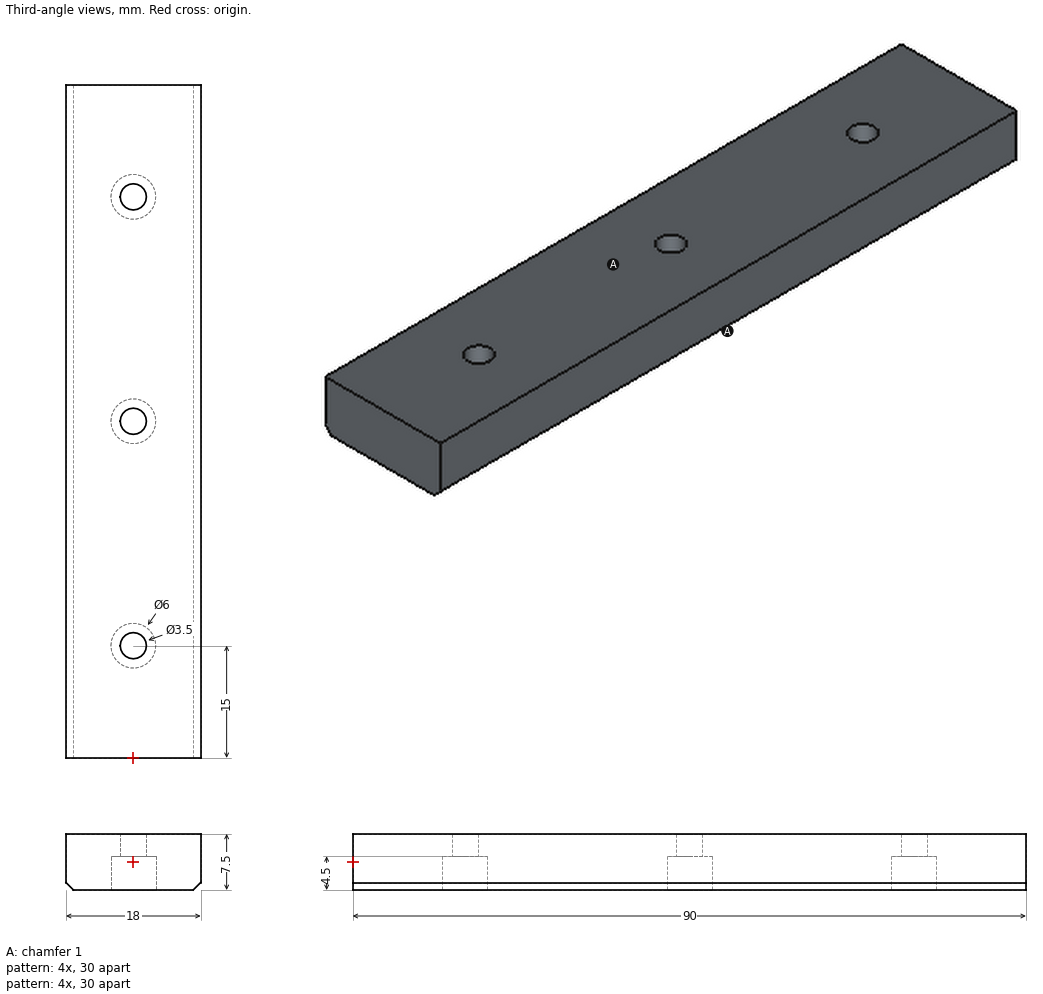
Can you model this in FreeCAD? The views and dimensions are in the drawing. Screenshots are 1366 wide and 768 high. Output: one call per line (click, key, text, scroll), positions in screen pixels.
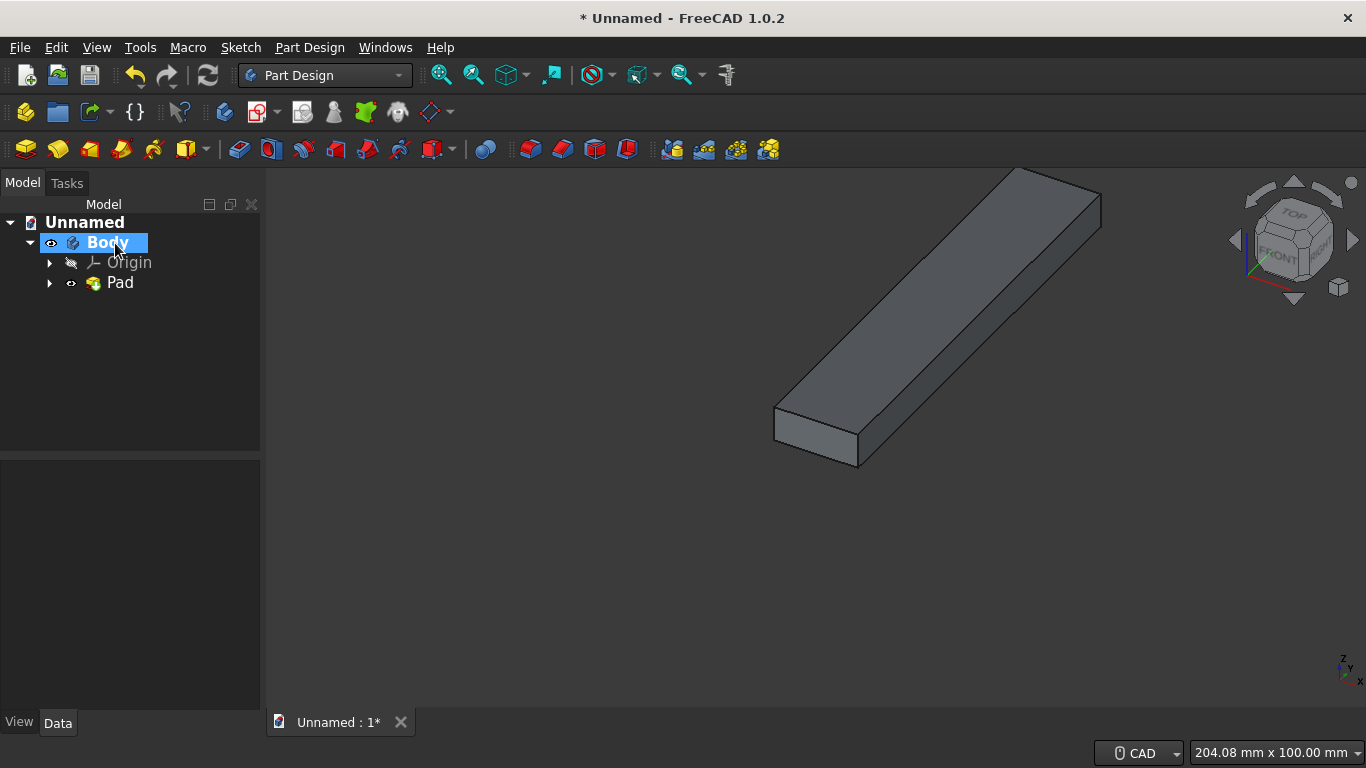
click(442, 76)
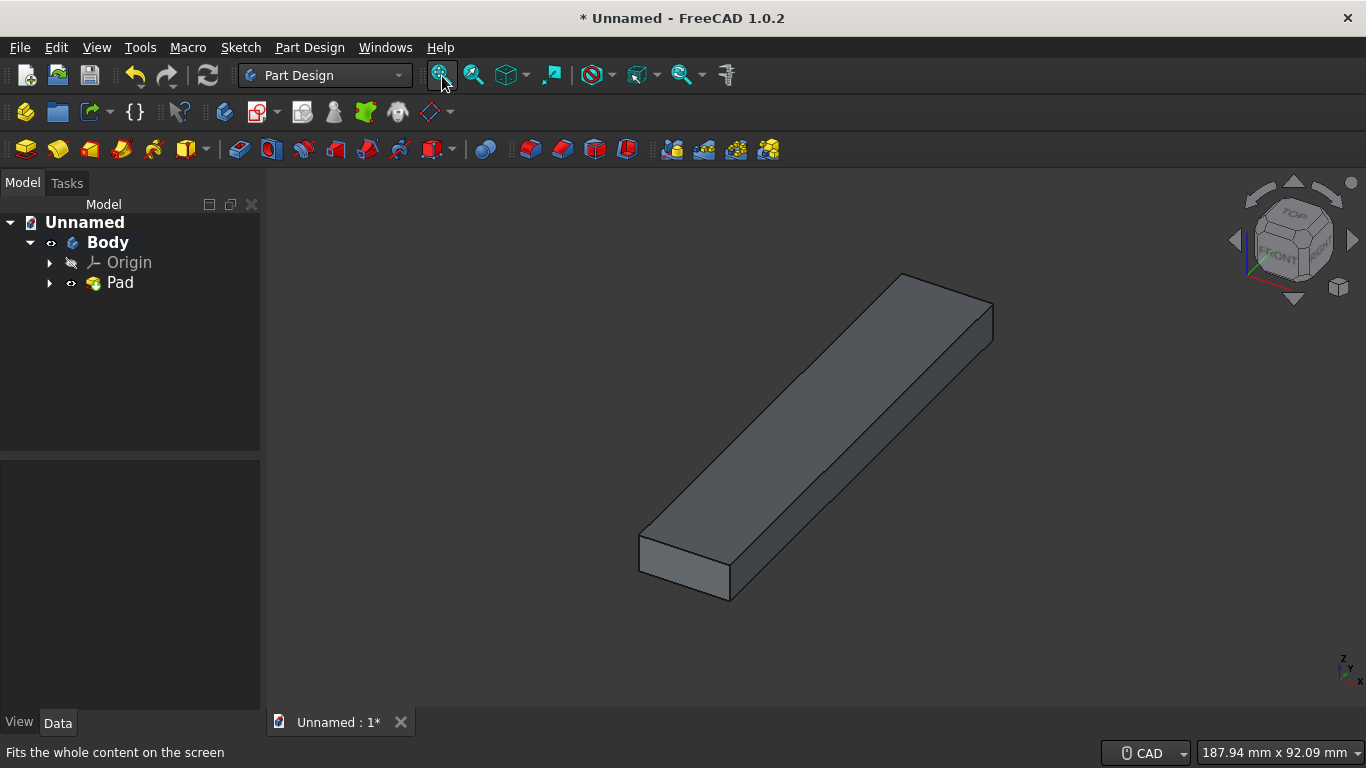
key(0)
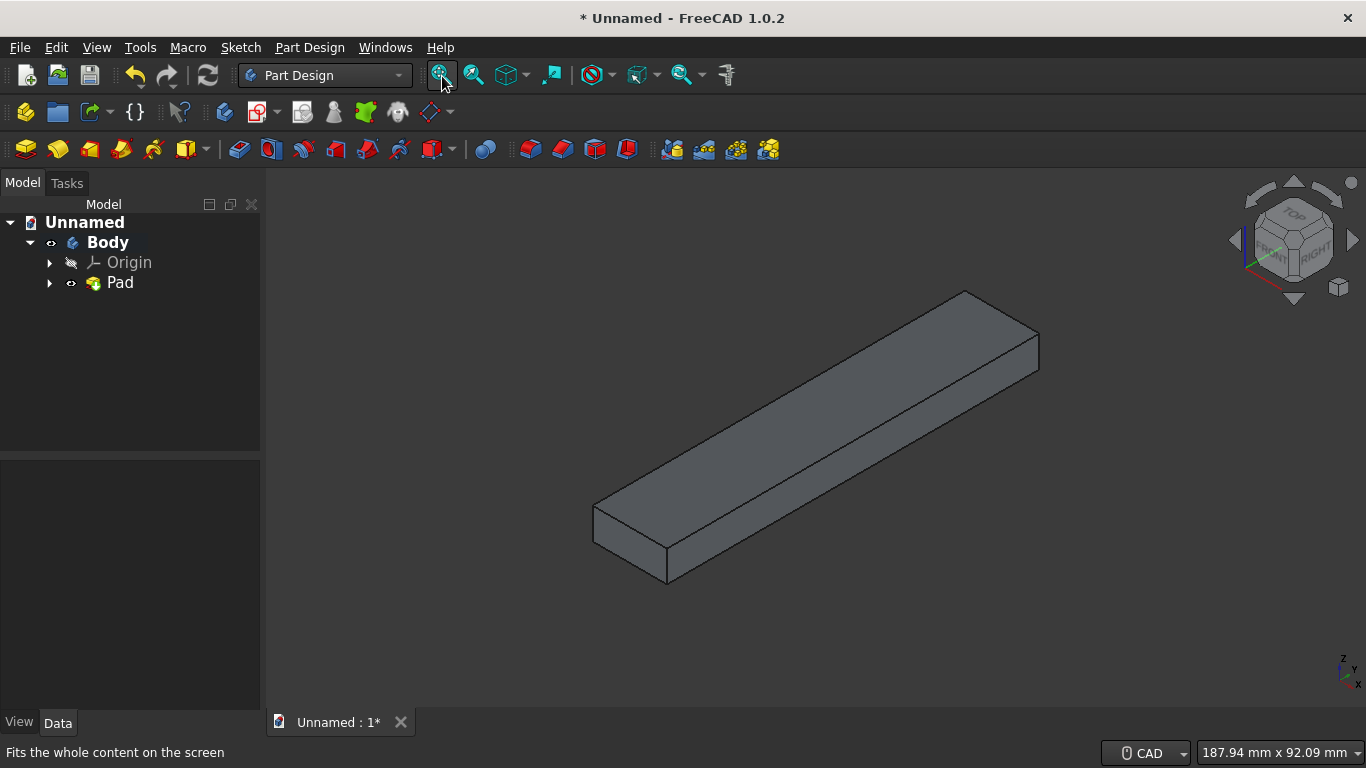
key(2)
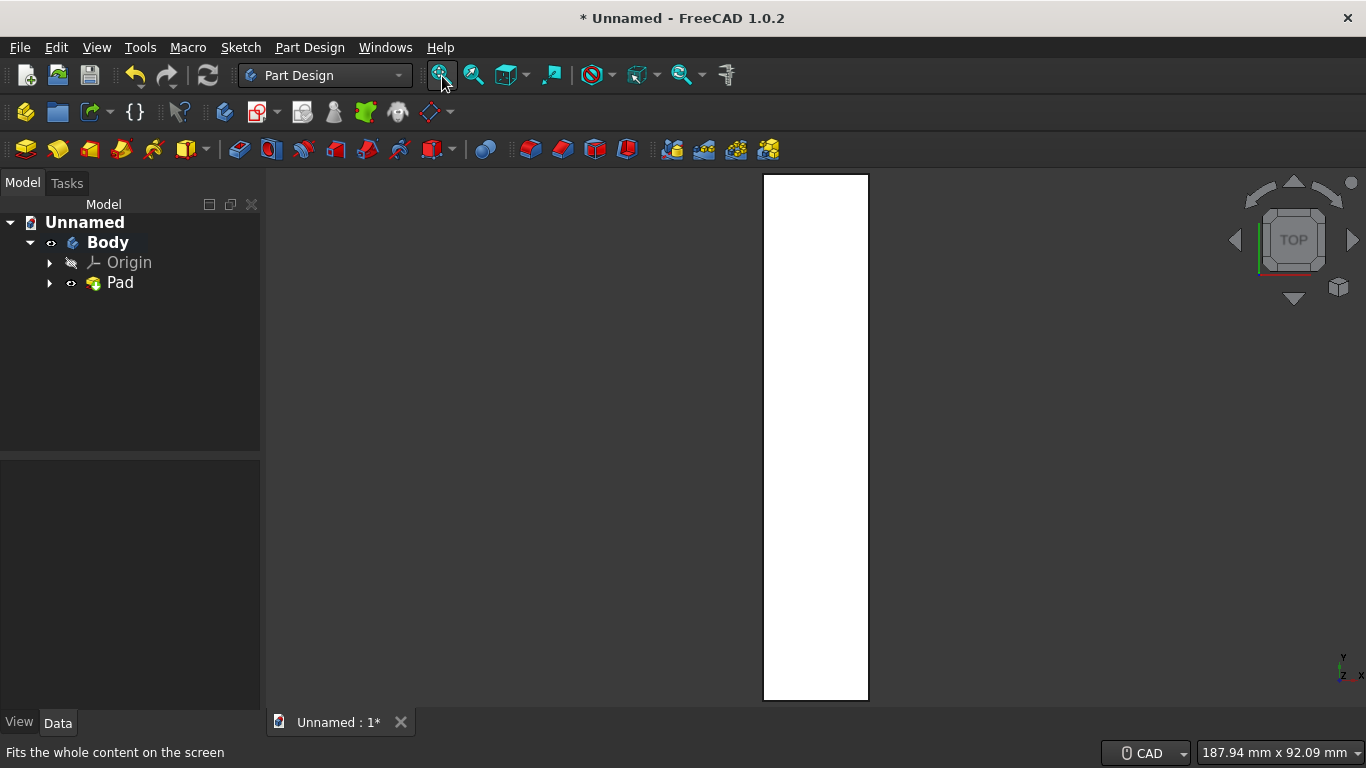
key(1)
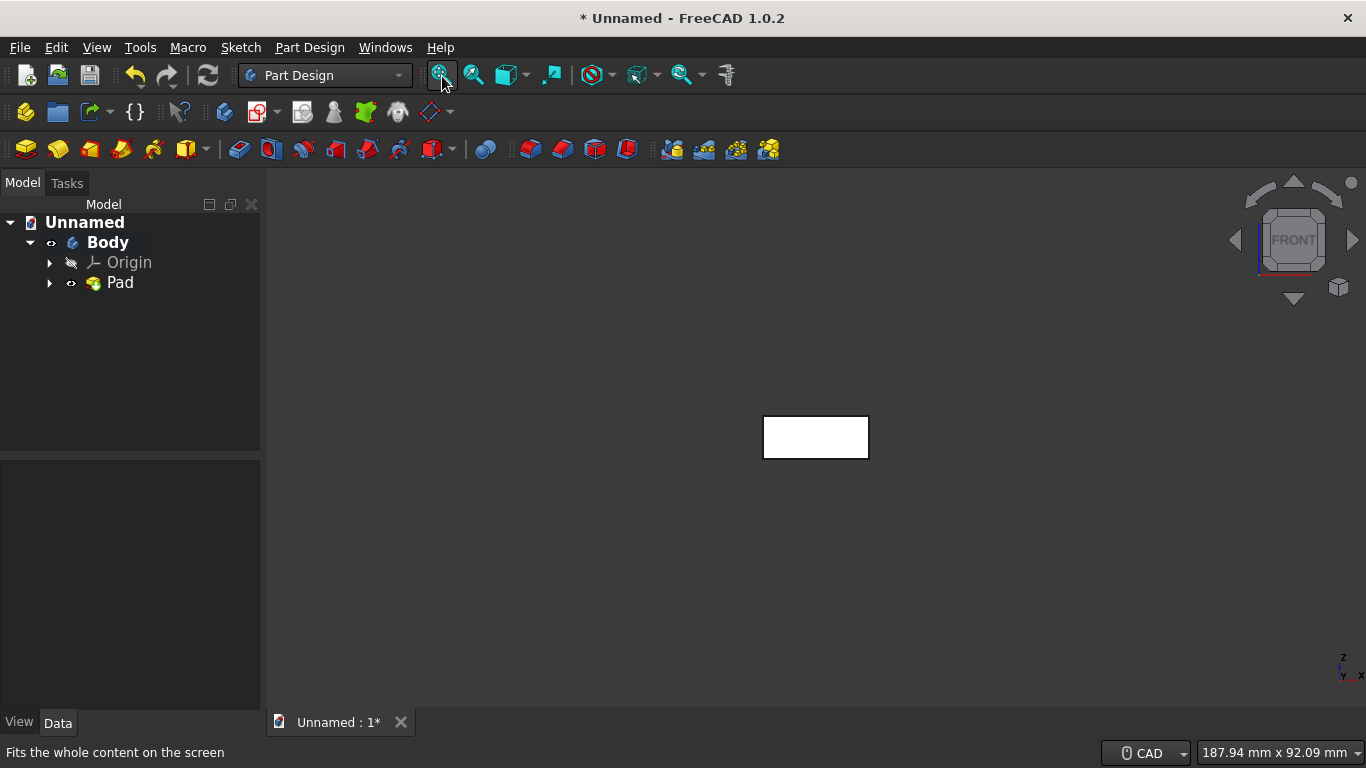
click(442, 76)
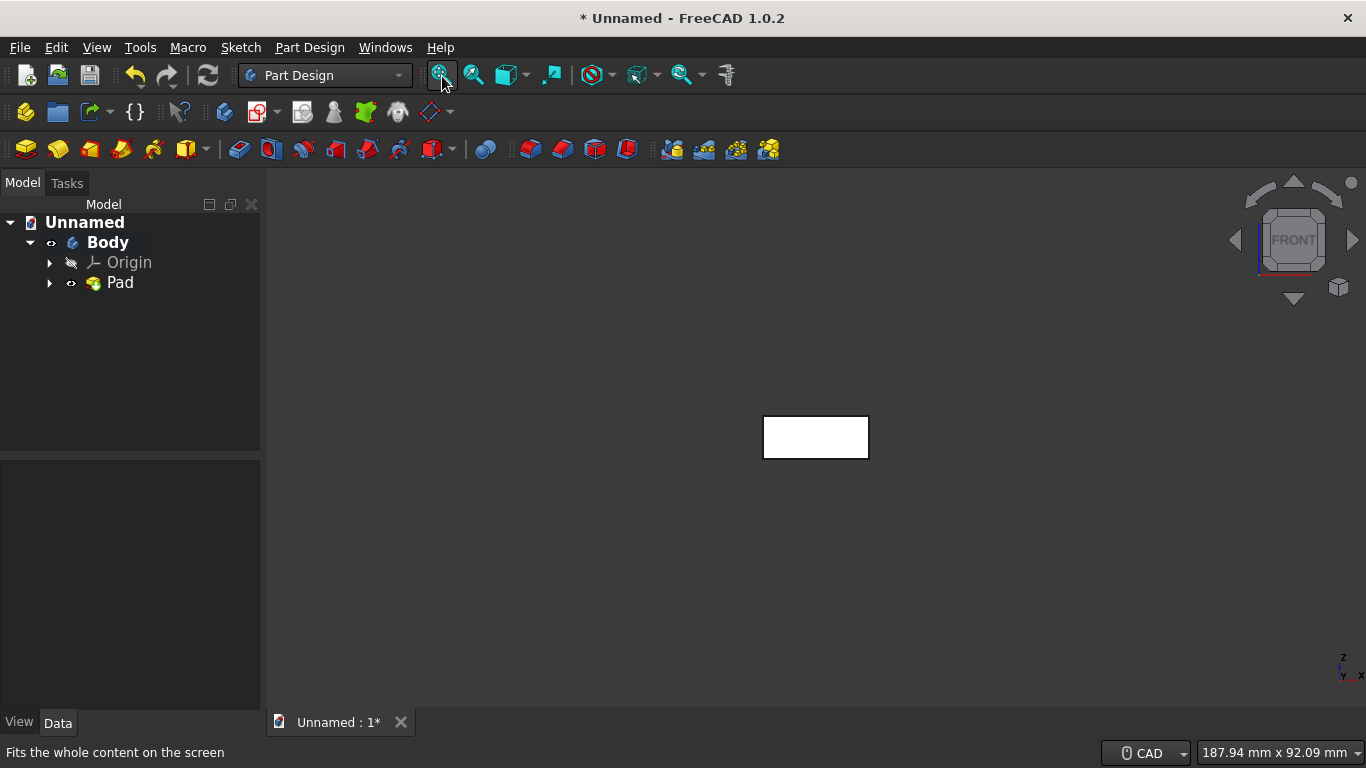
key(3)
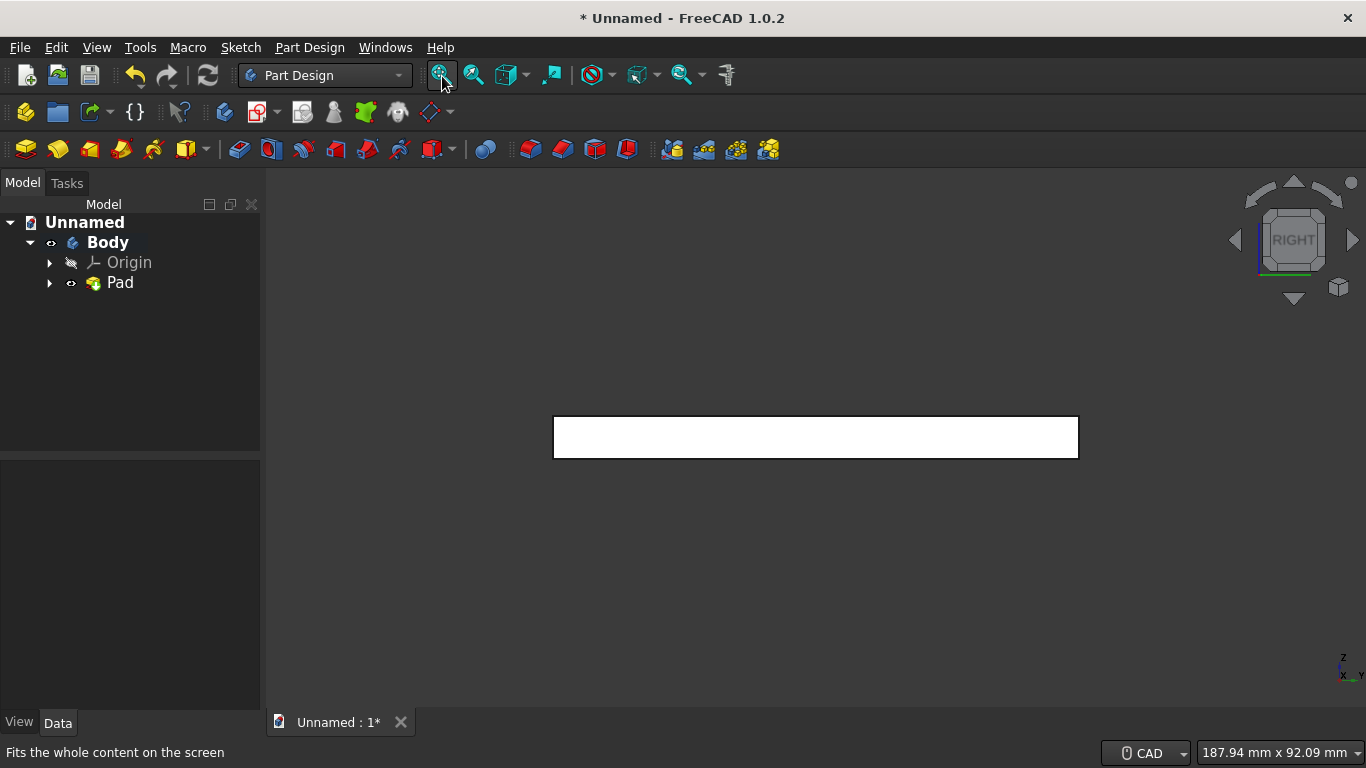
click(816, 458)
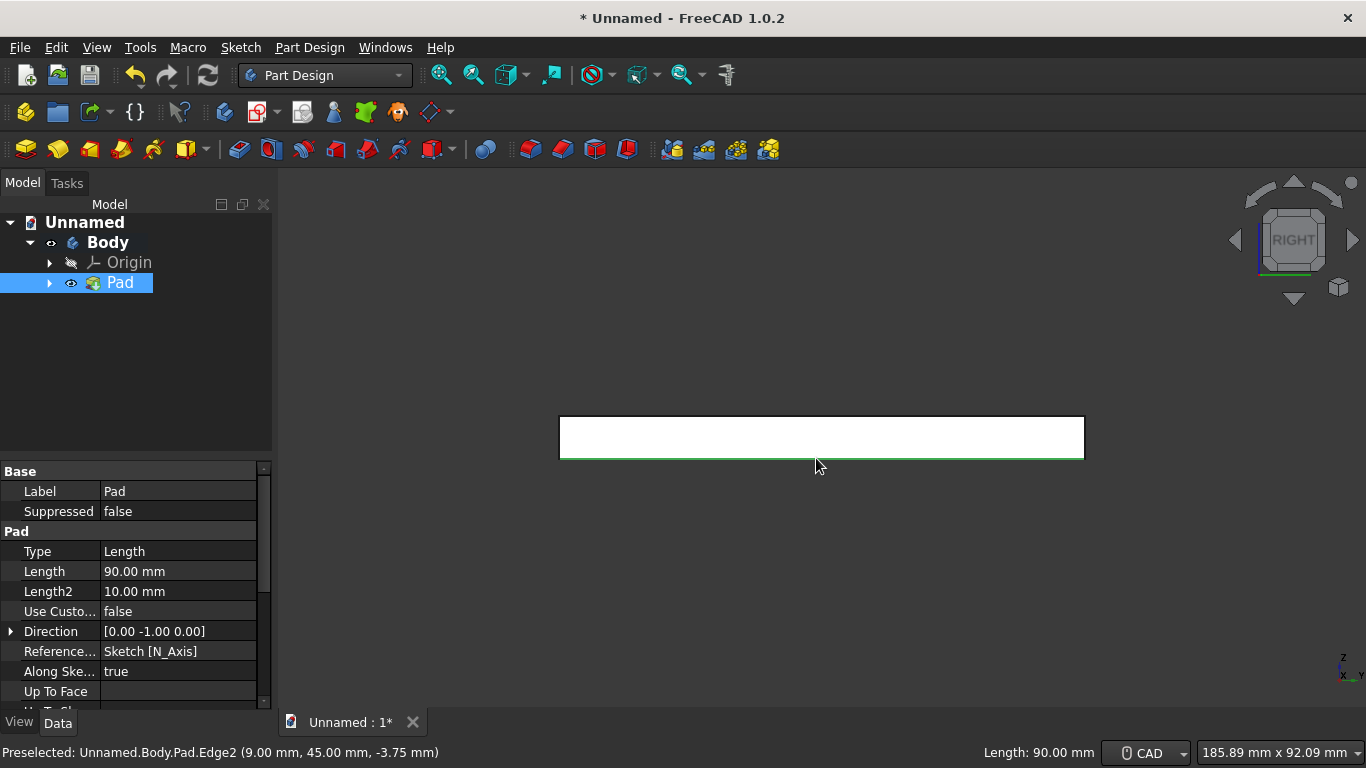
key(5)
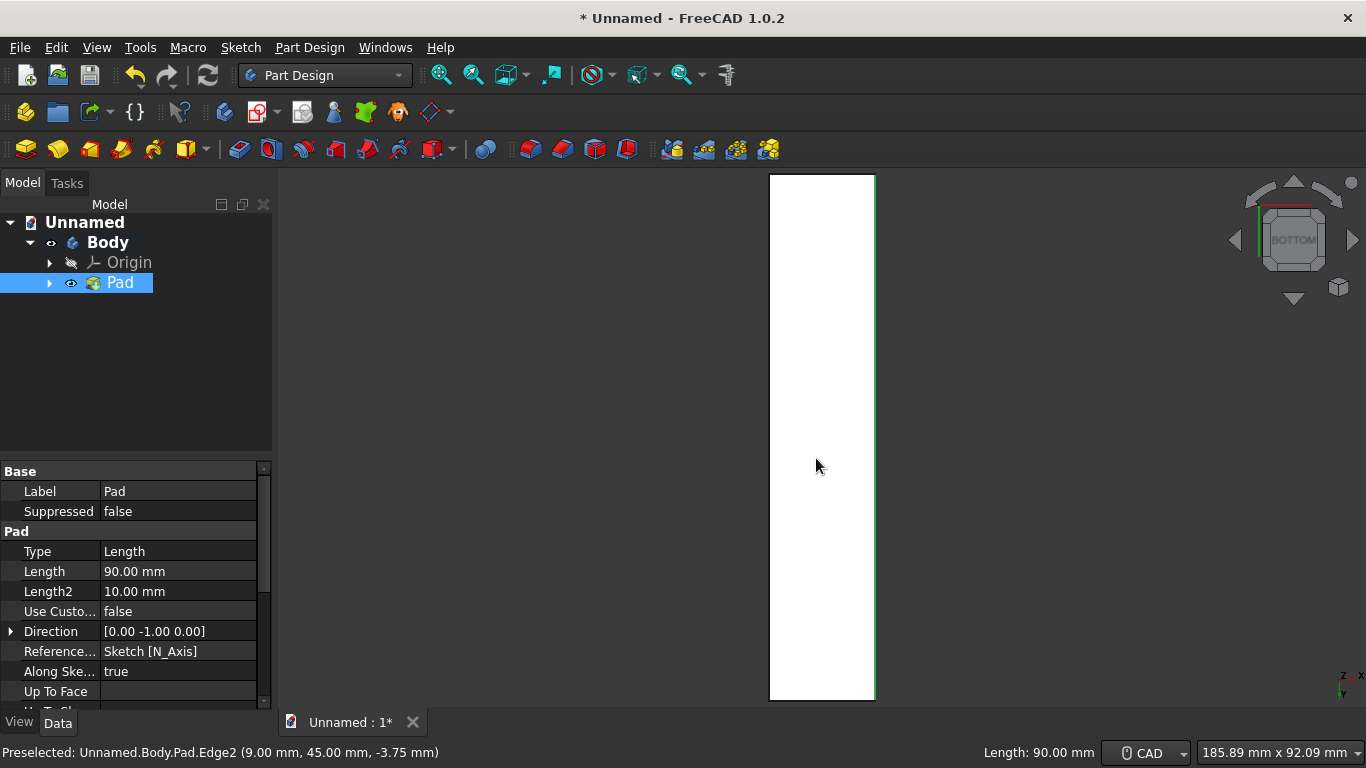
click(769, 436, ctrl)